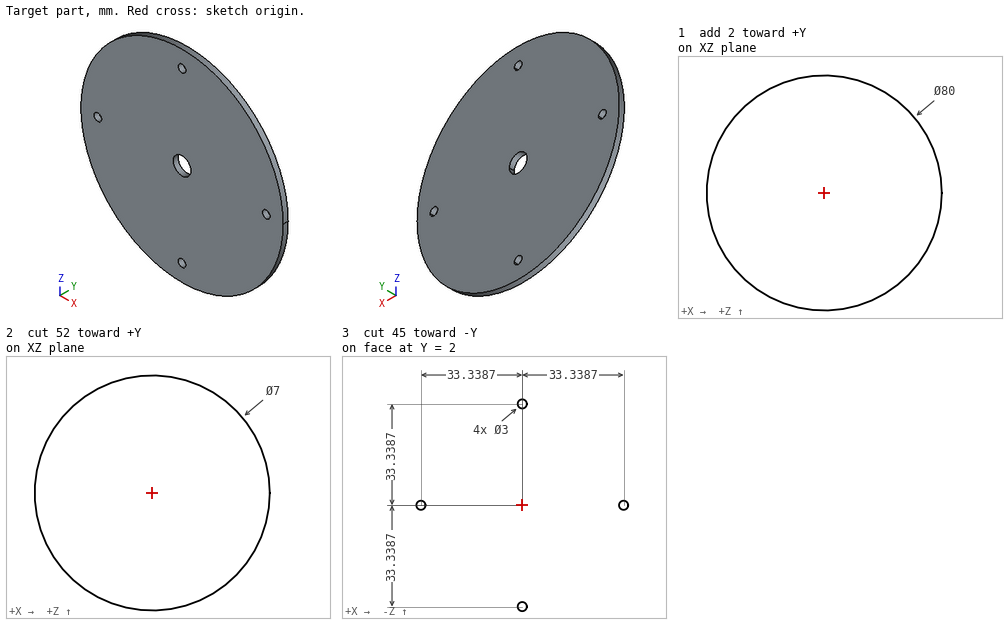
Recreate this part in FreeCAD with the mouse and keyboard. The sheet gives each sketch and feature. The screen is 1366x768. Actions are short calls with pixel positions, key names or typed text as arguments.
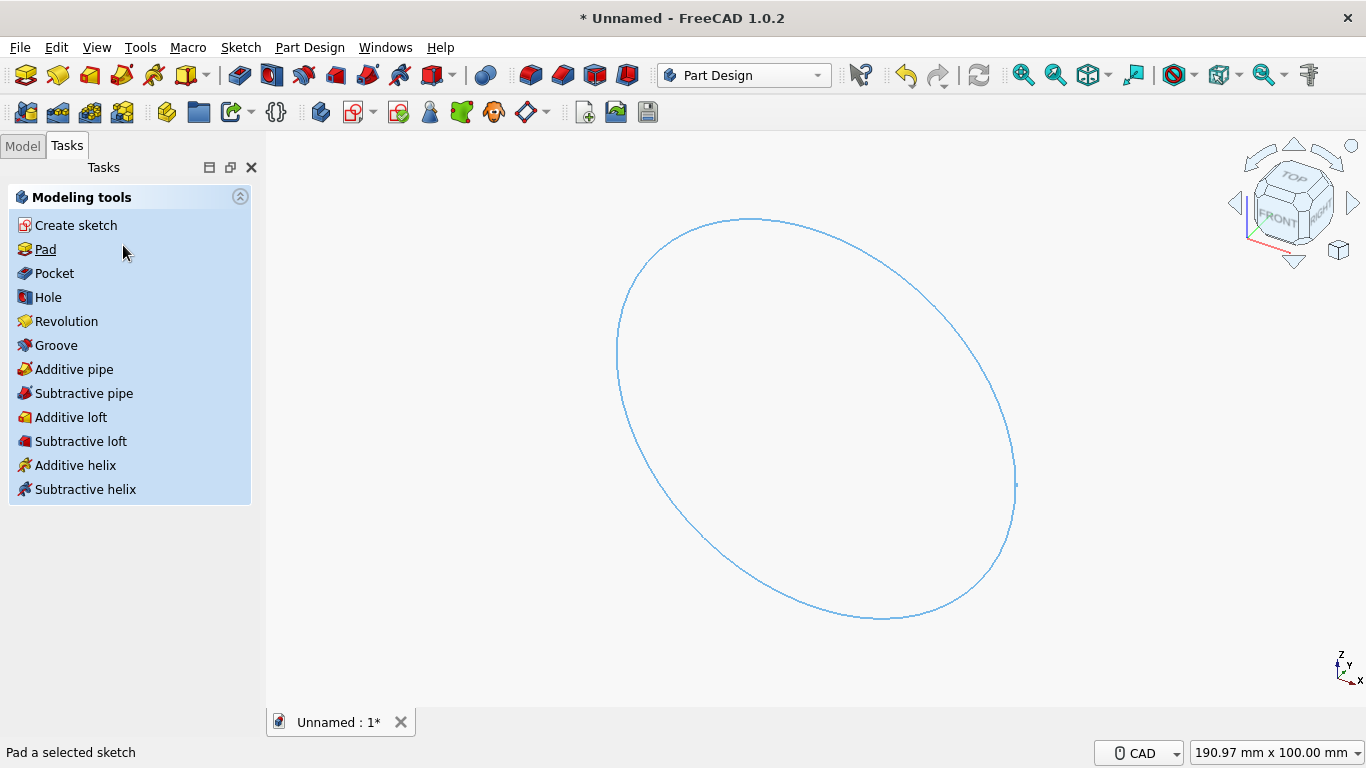
click(26, 76)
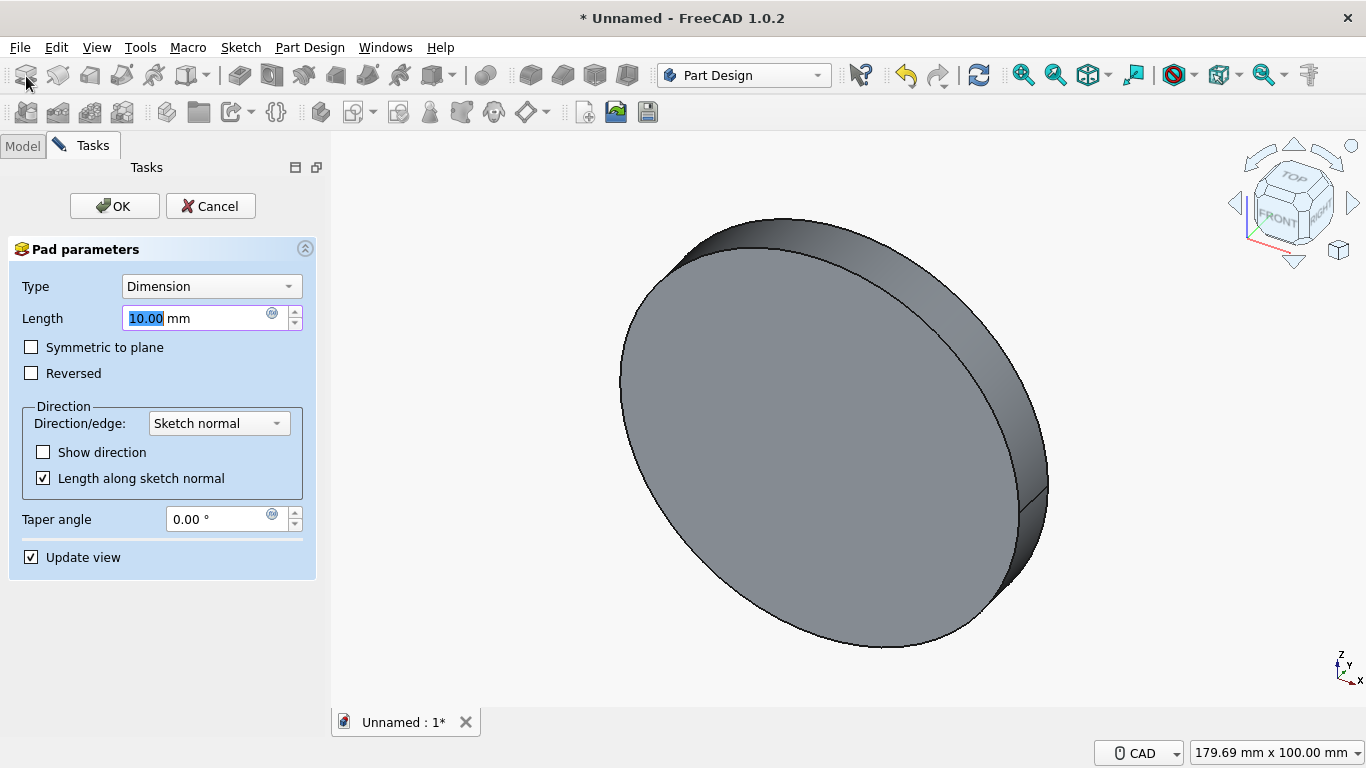
text(2)
key(Tab)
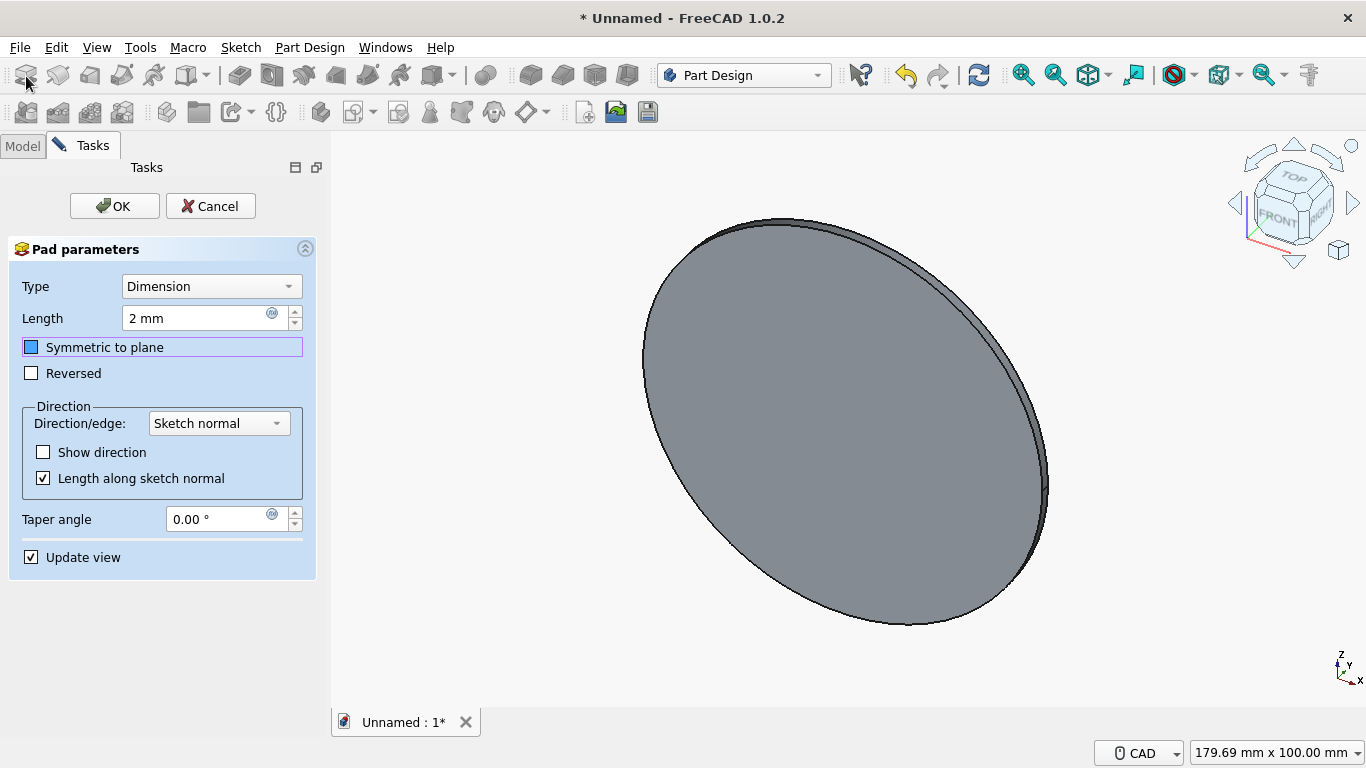
click(30, 373)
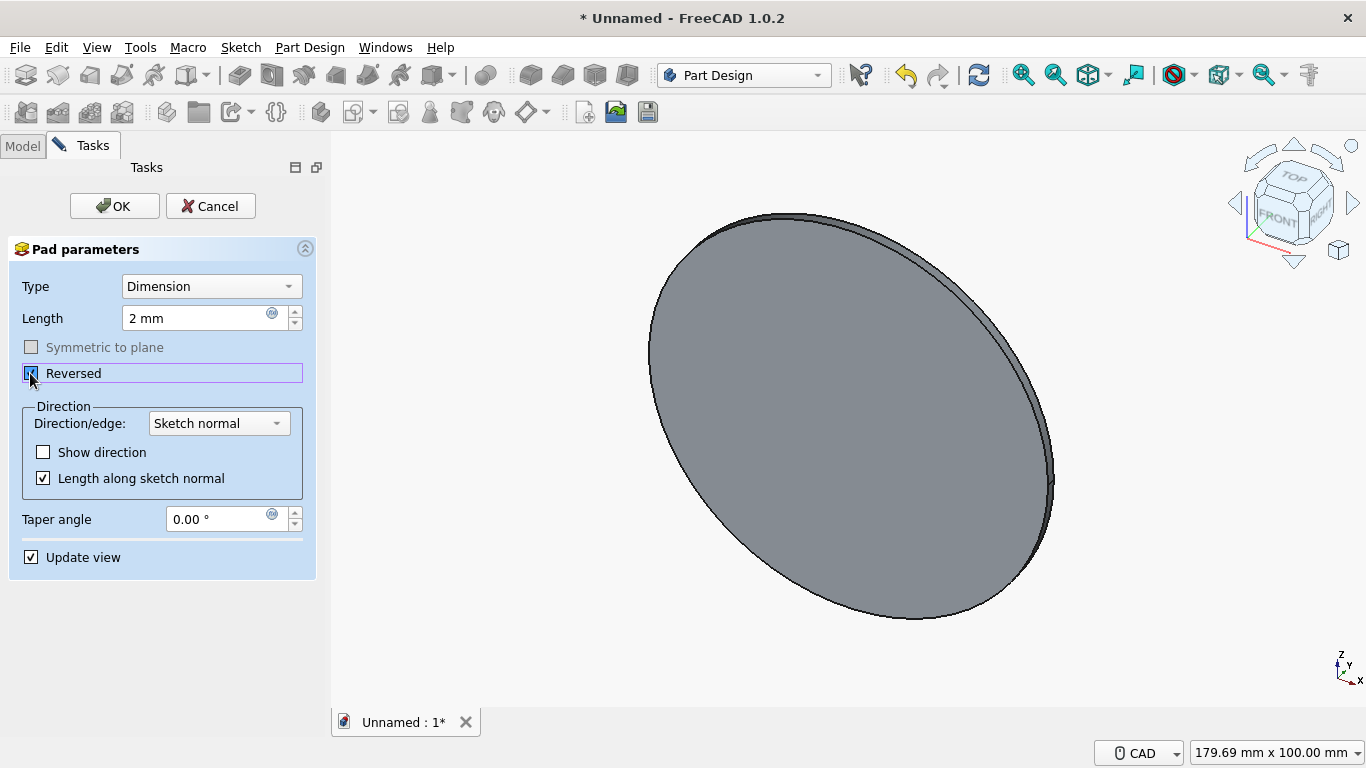
click(115, 206)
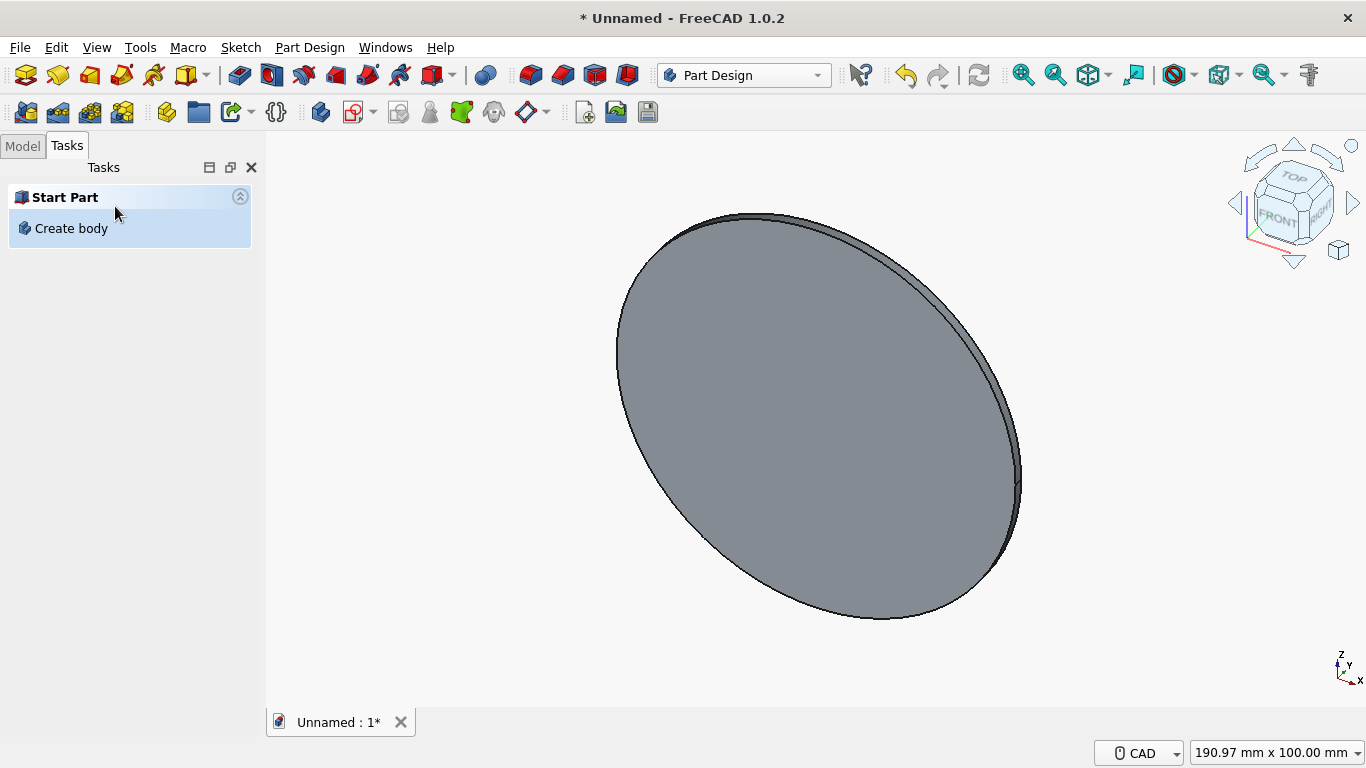
click(354, 112)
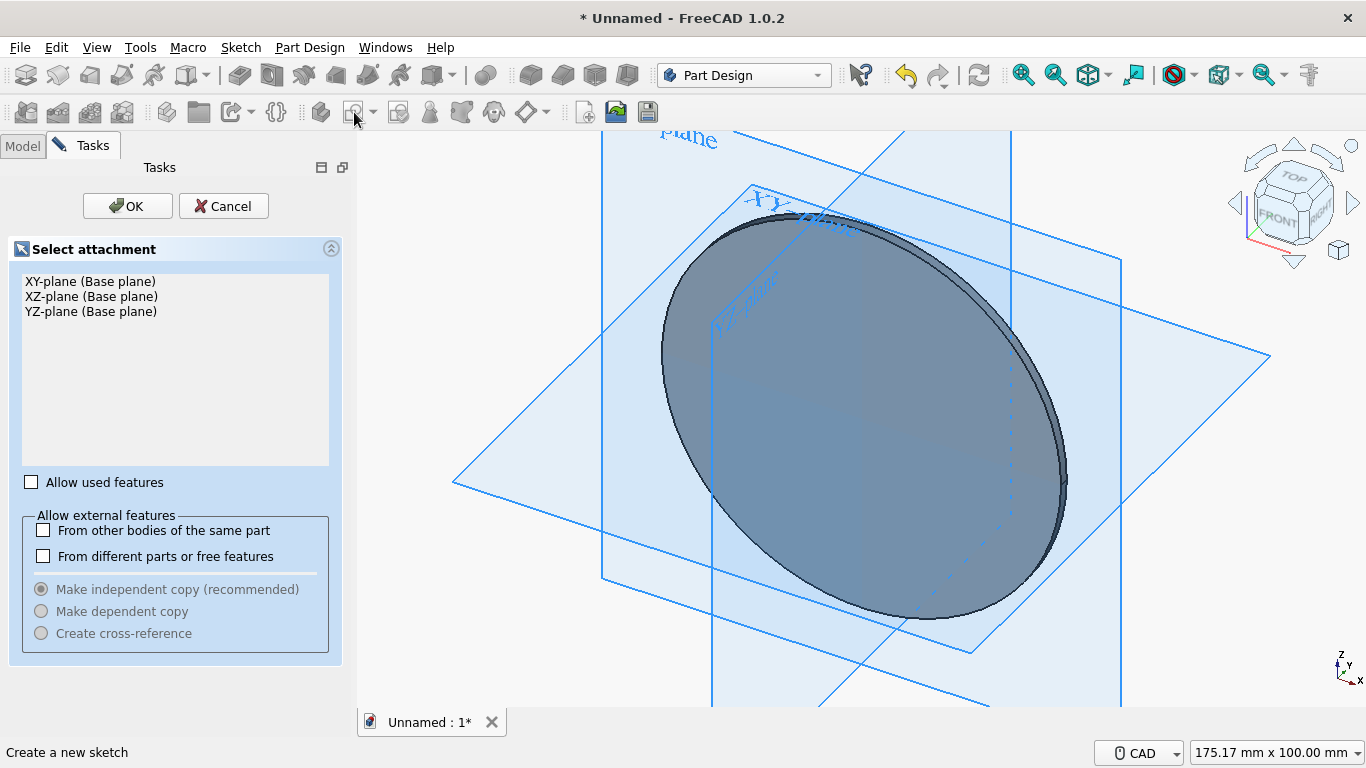
click(82, 296)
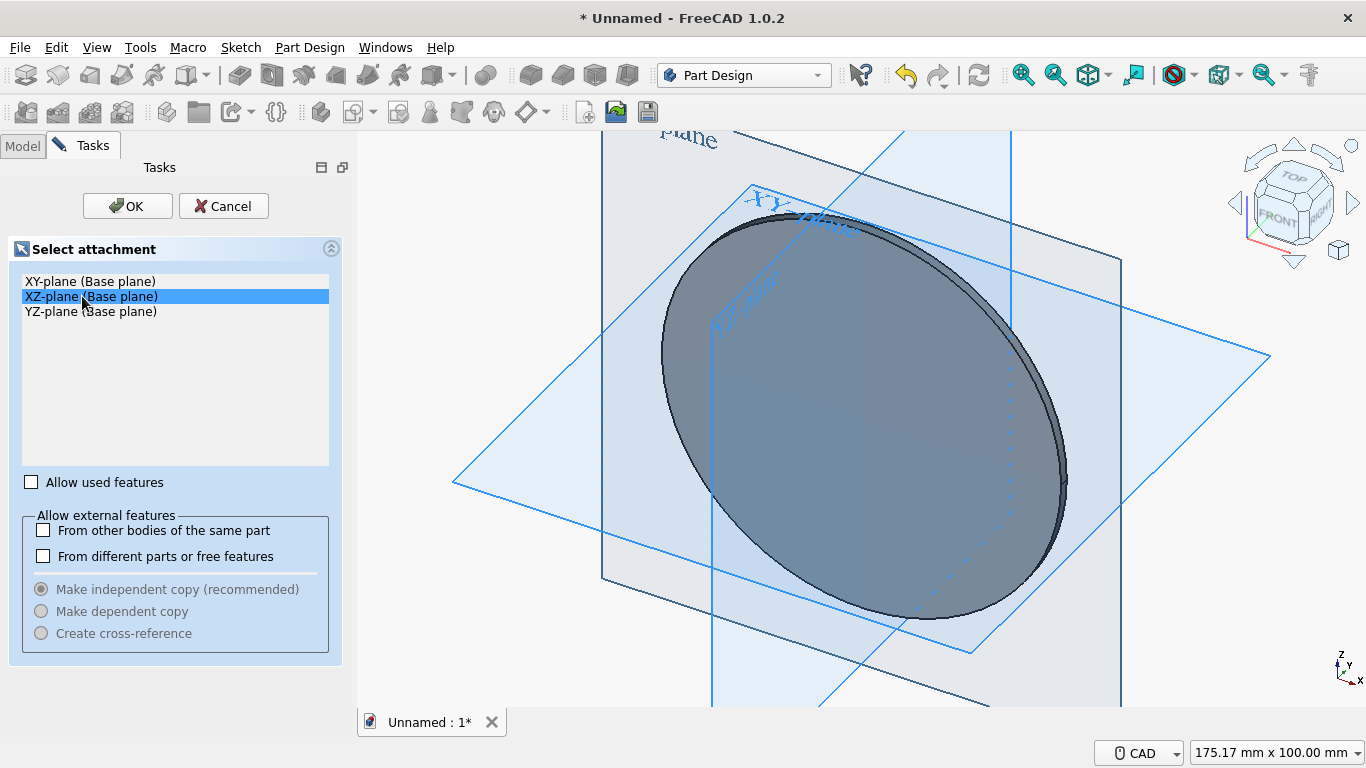
click(128, 206)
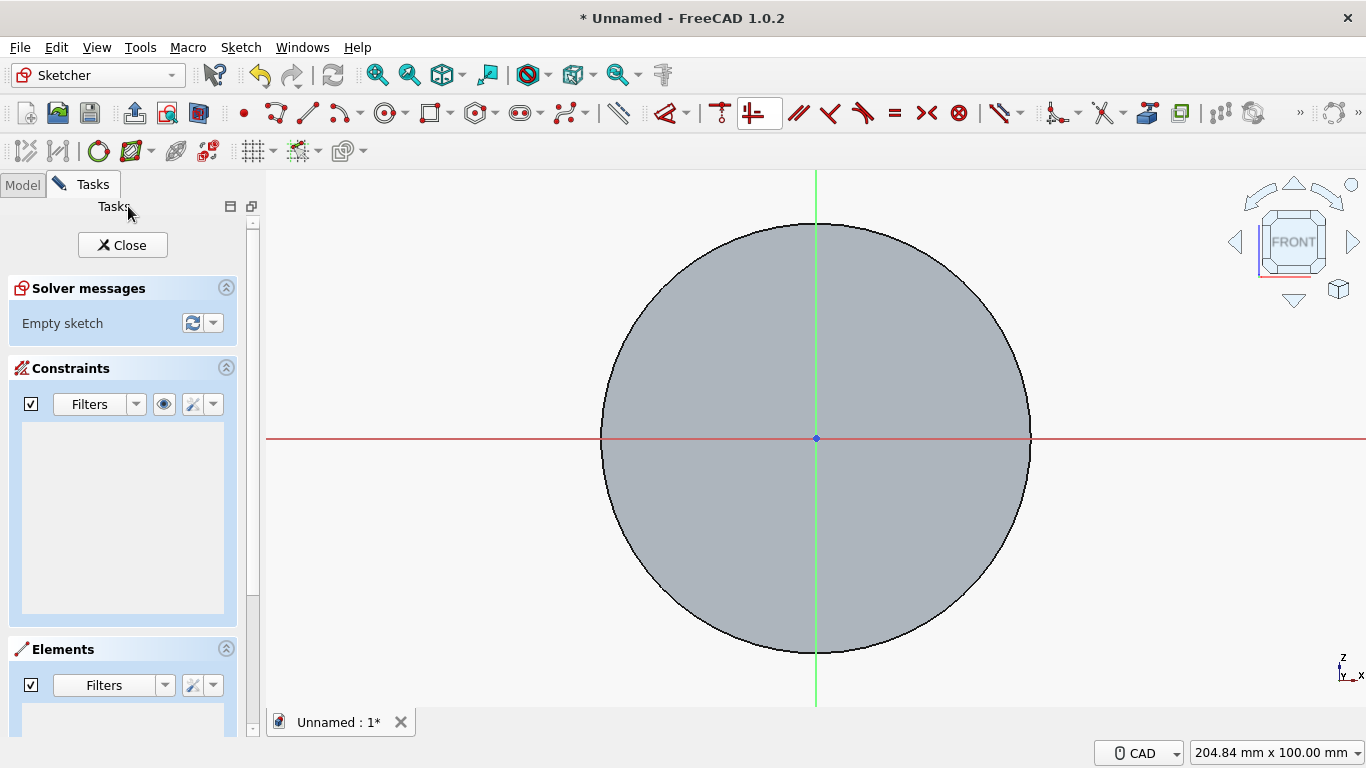
scroll(825, 438, up, 11)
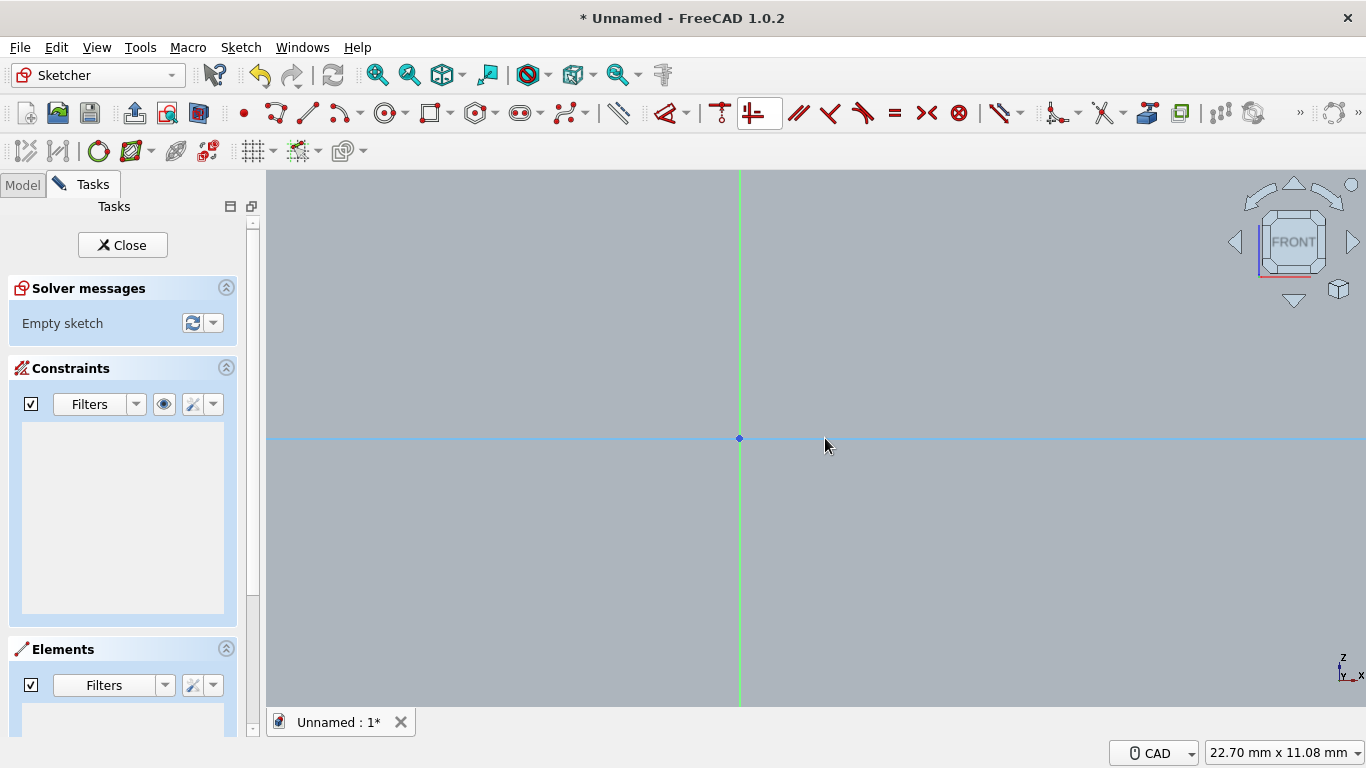
click(386, 114)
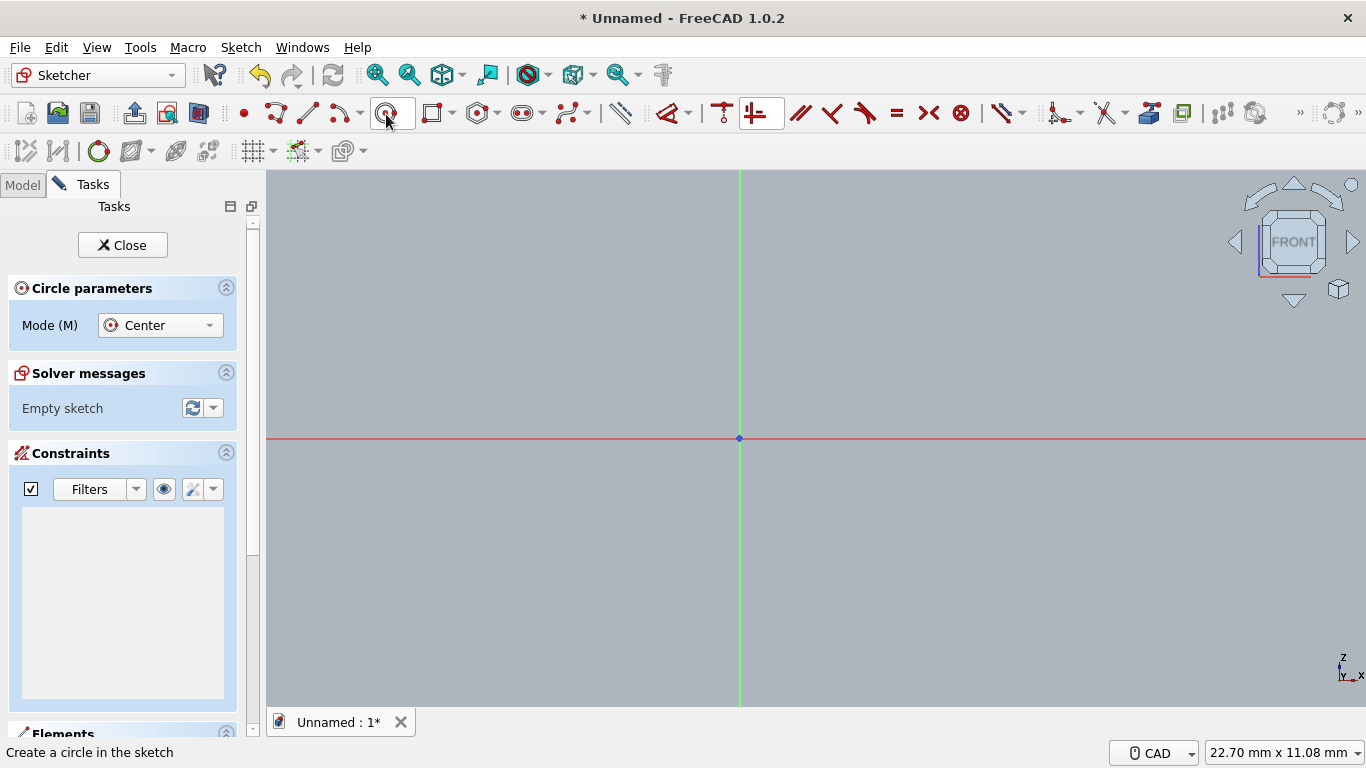
click(740, 438)
click(860, 319)
key(Escape)